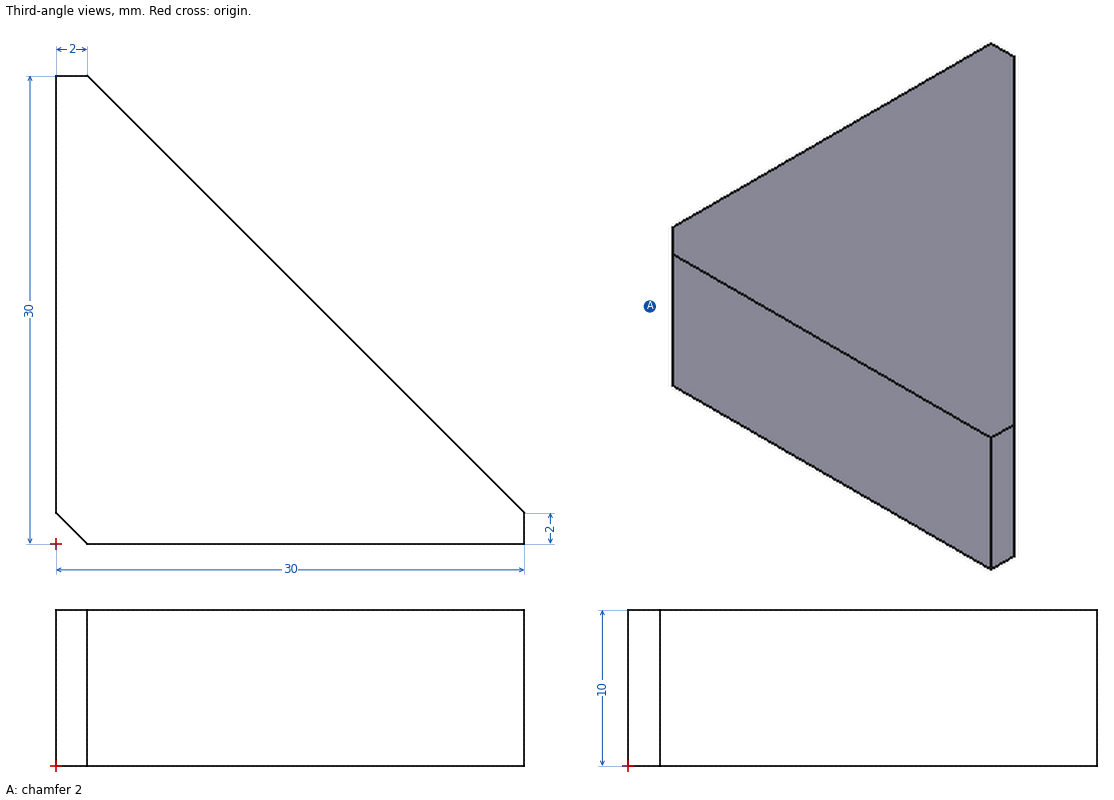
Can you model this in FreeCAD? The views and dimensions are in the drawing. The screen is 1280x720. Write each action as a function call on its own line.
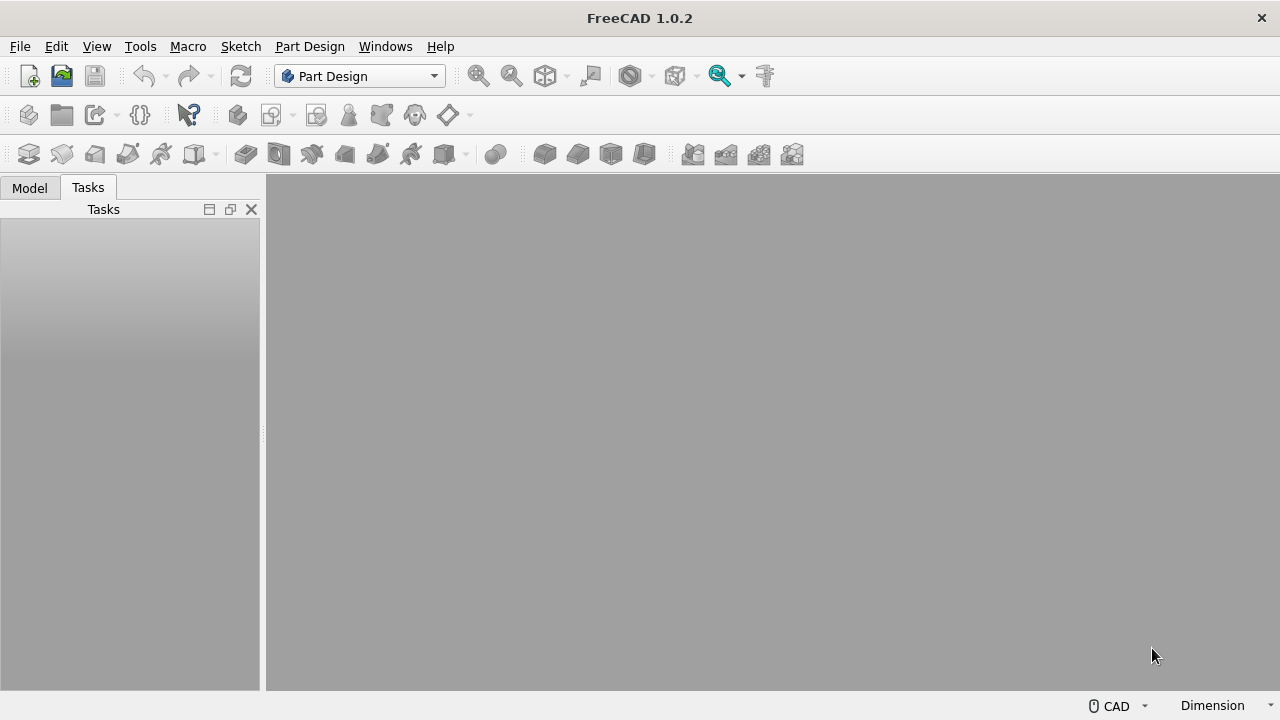
click(29, 76)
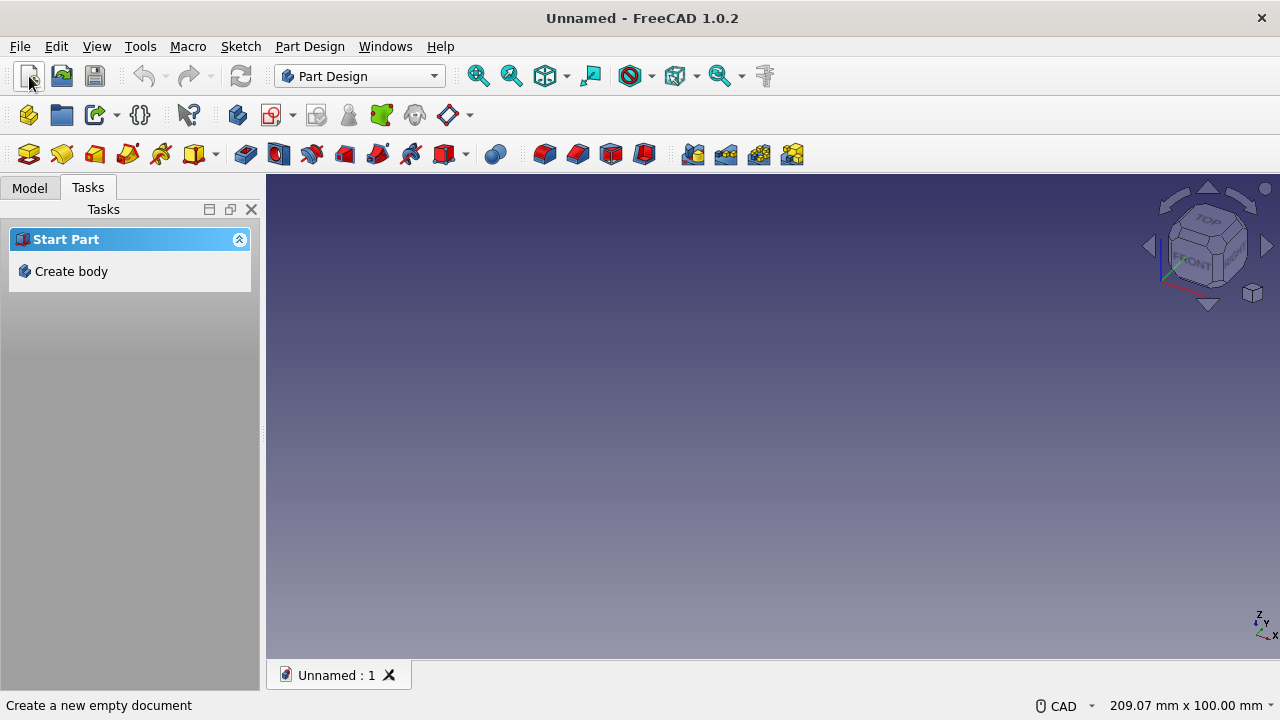
click(270, 116)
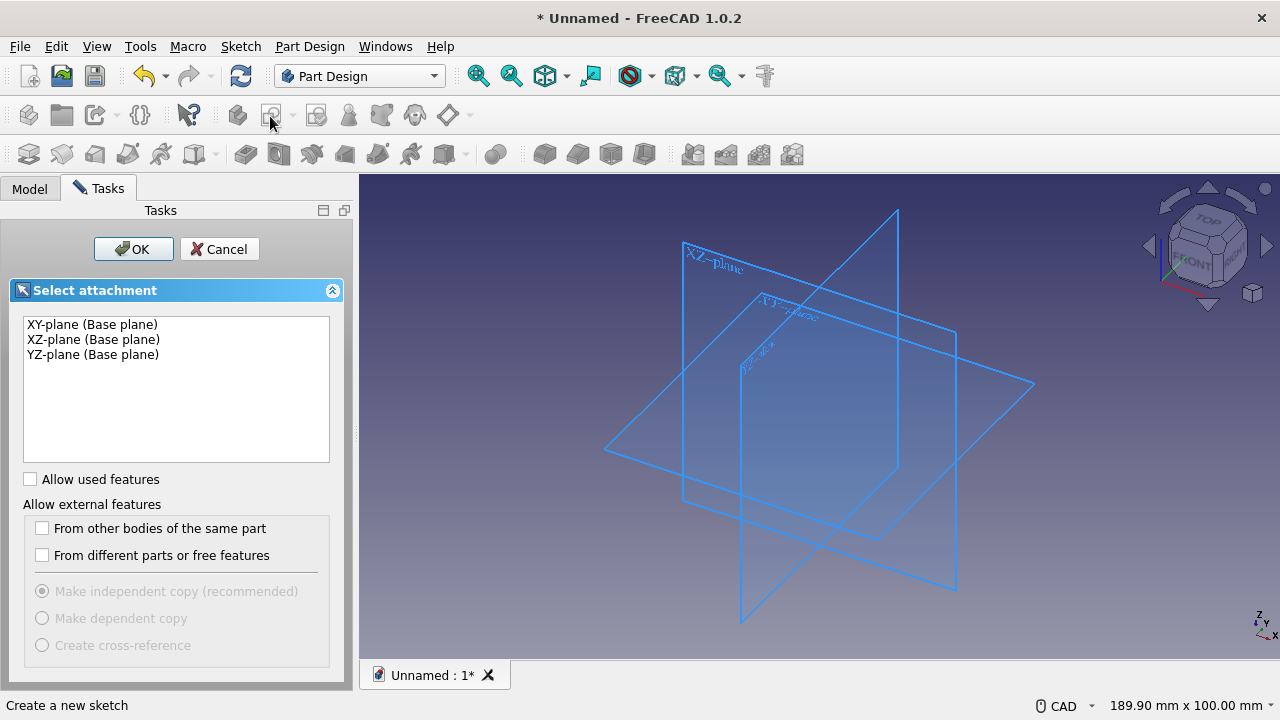
click(84, 324)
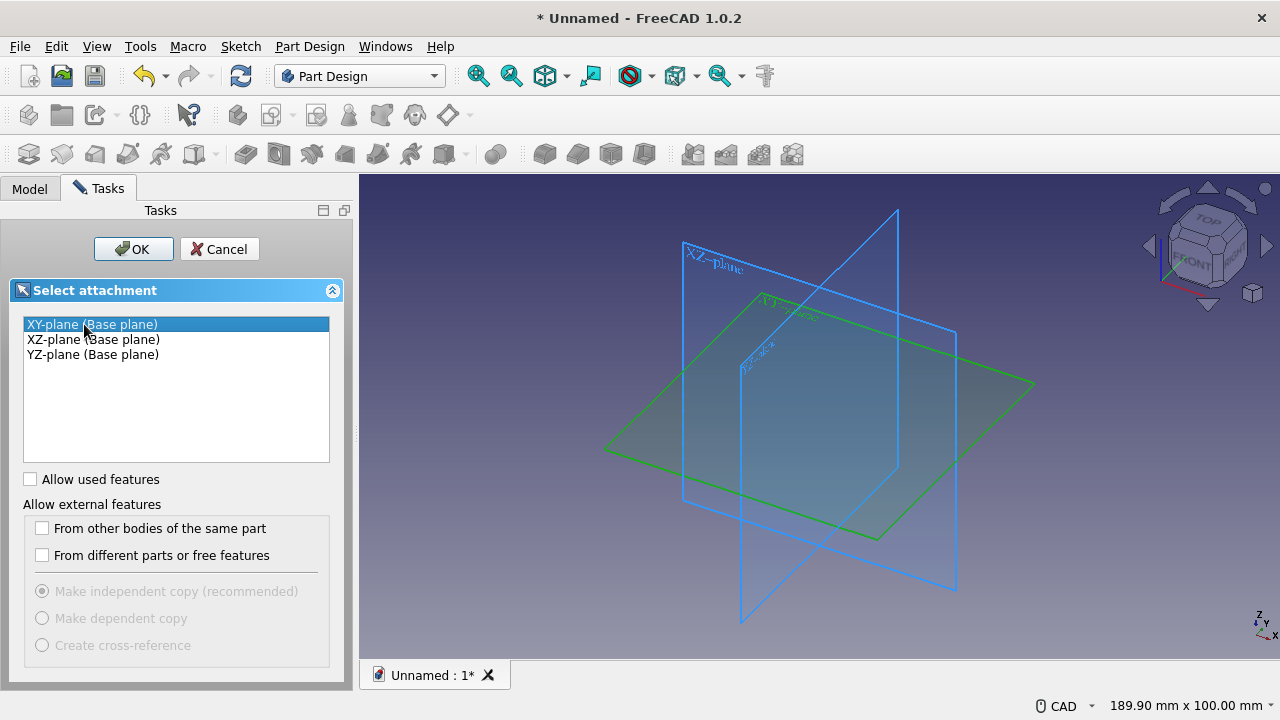
click(134, 249)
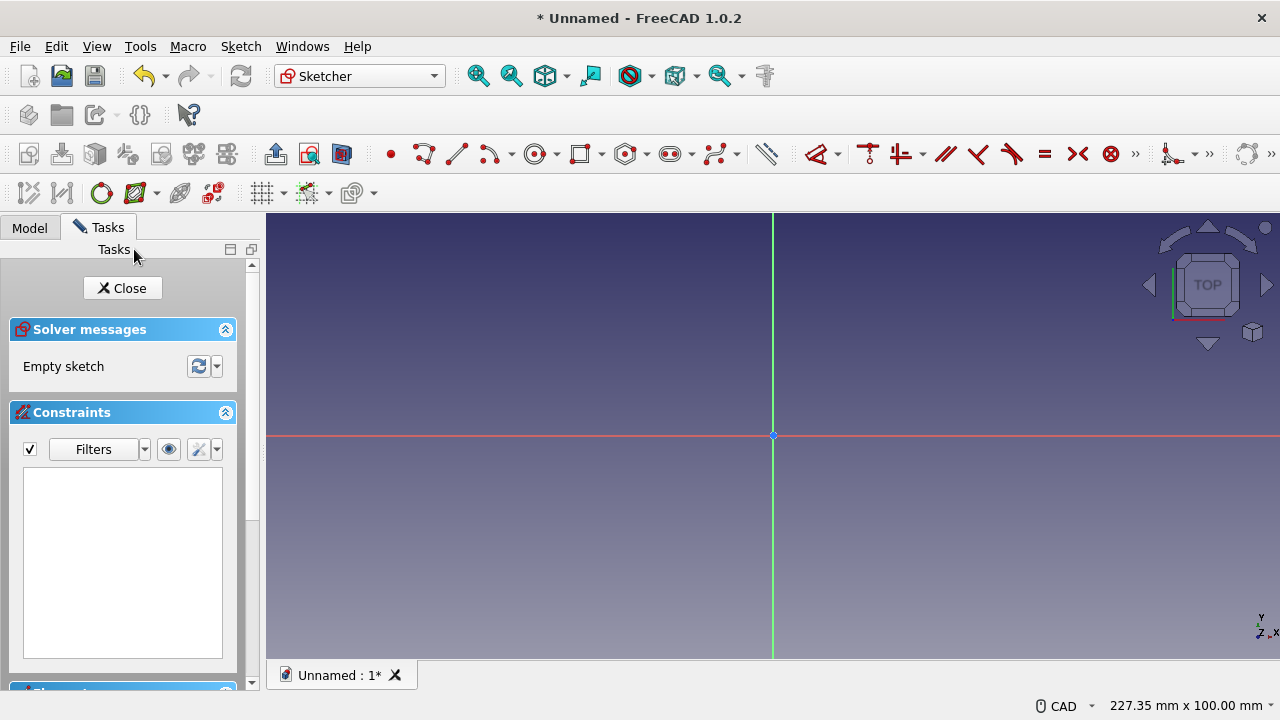
scroll(950, 315, up, 4)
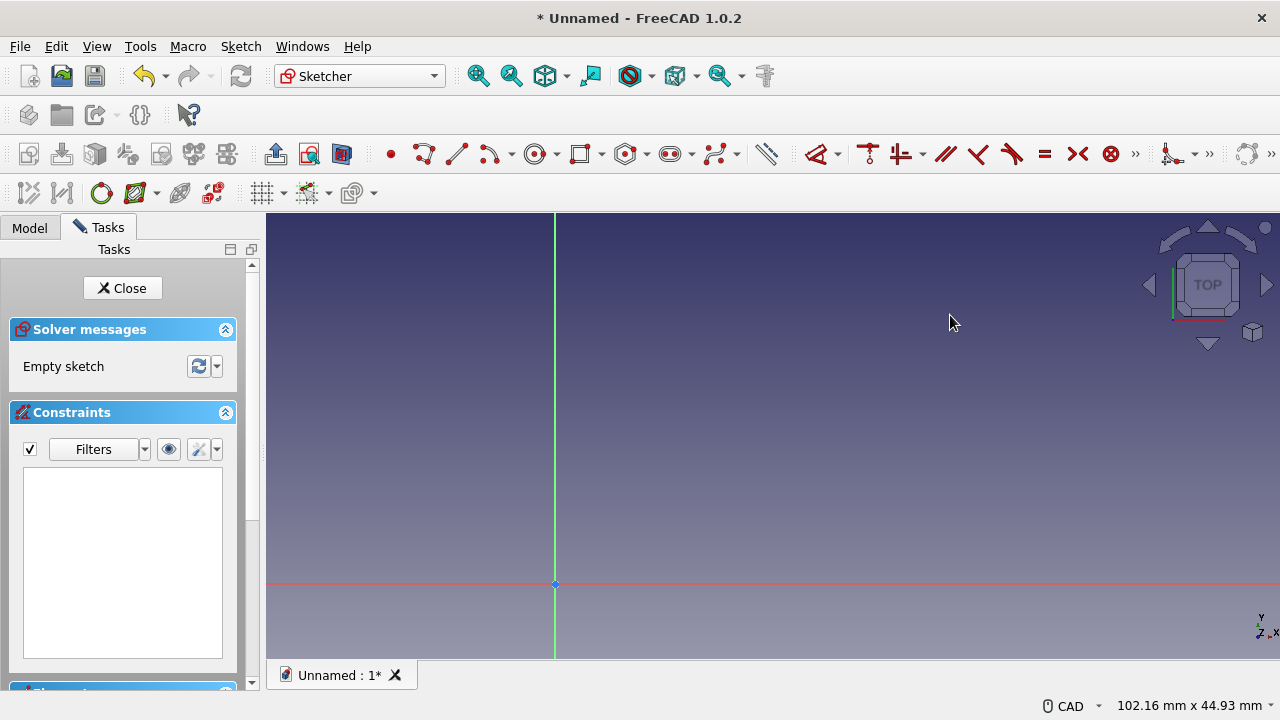
click(424, 154)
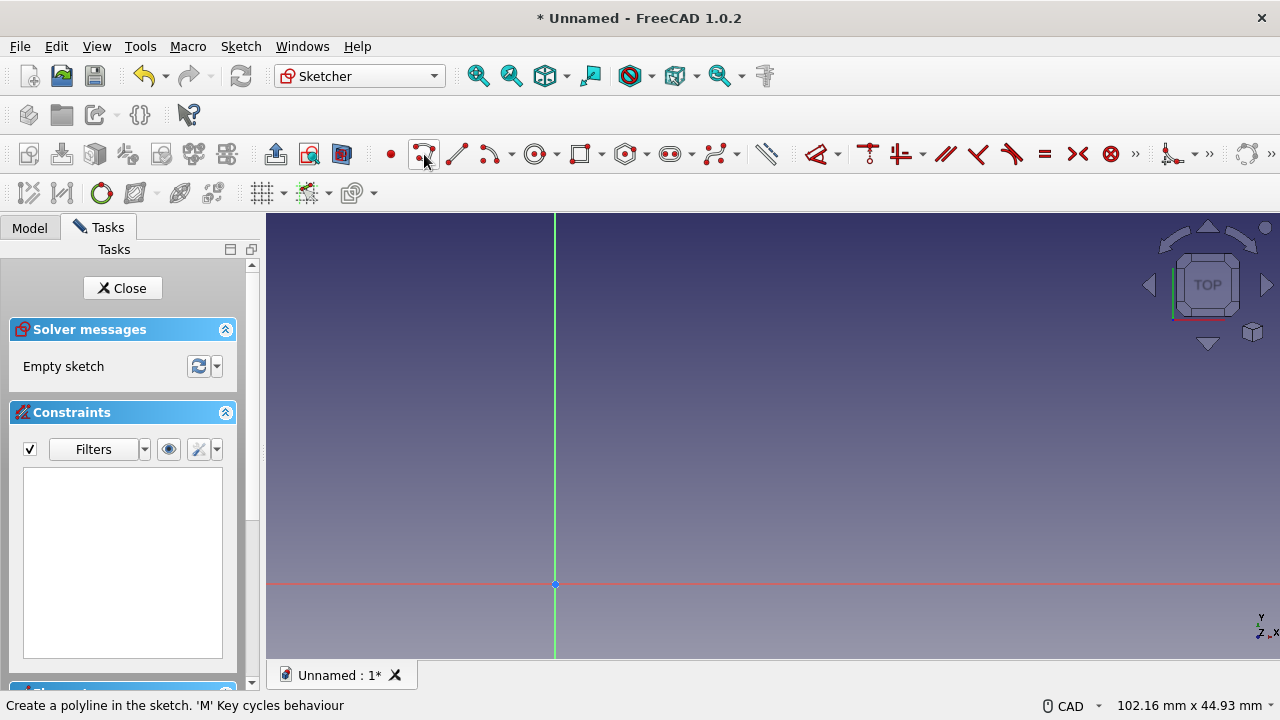
click(555, 584)
click(853, 575)
click(853, 564)
click(575, 286)
click(564, 286)
click(555, 584)
key(Escape)
key(Escape)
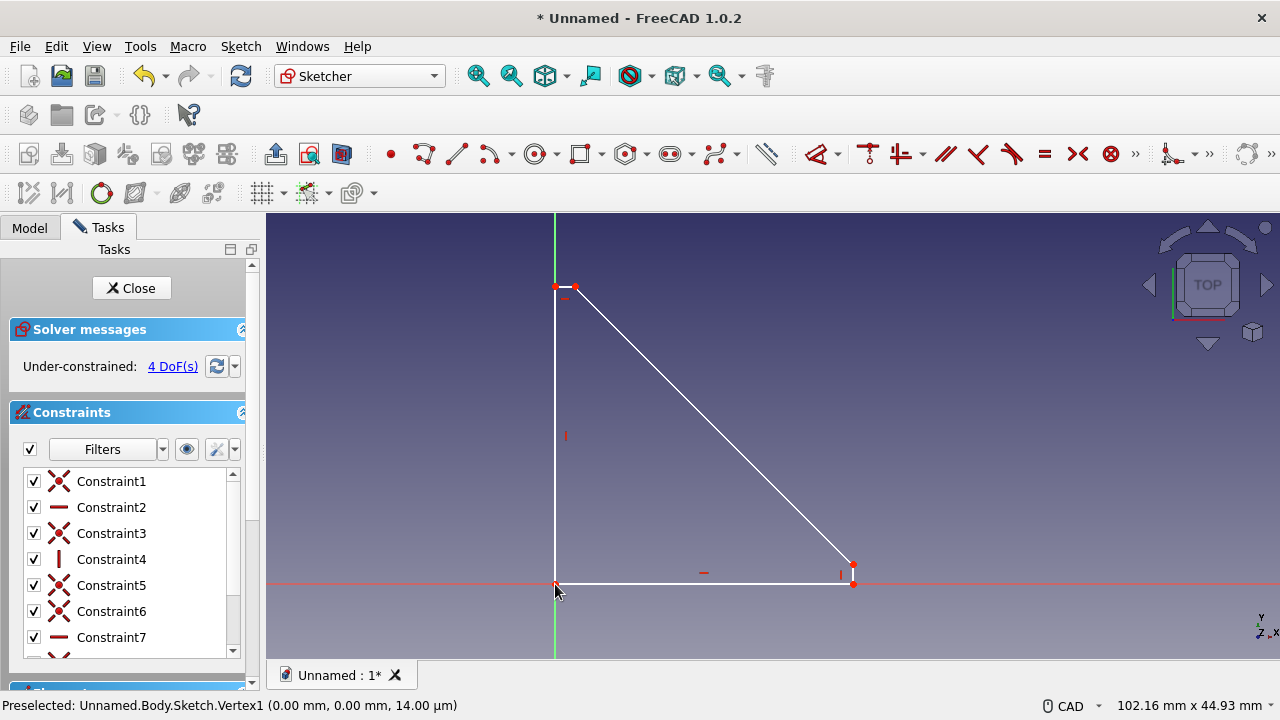
click(816, 154)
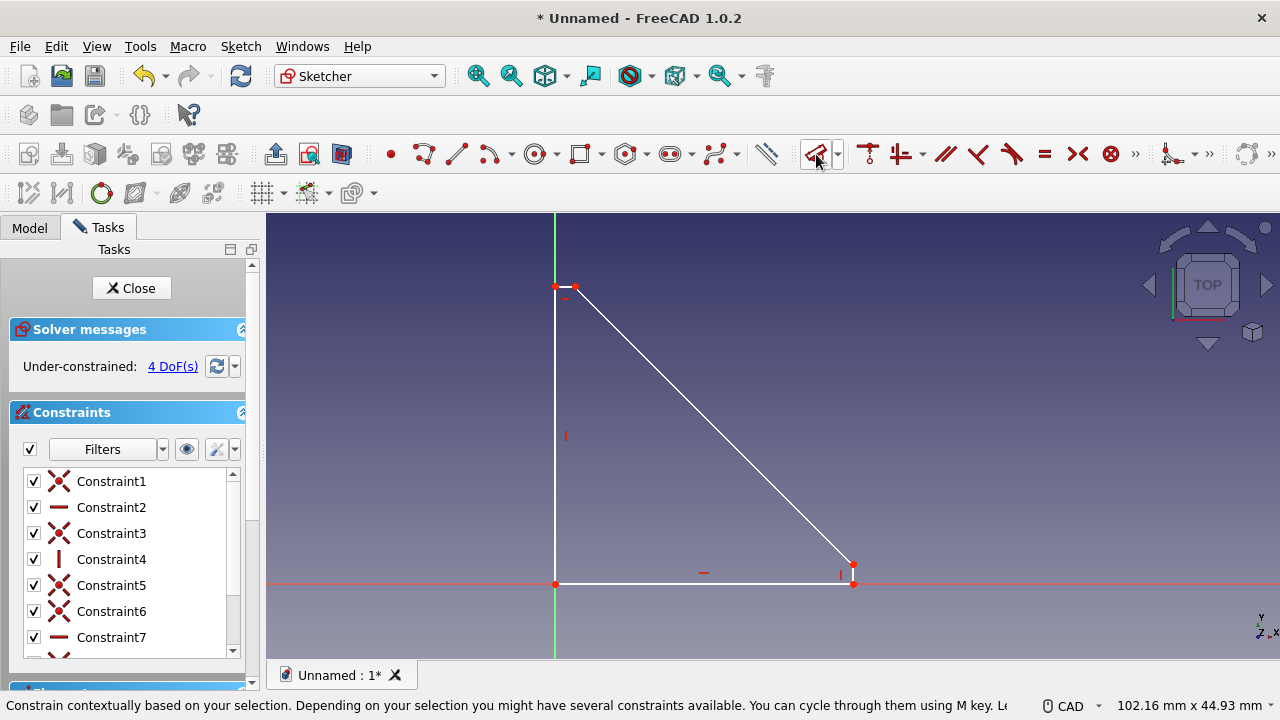
scroll(853, 575, up, 4)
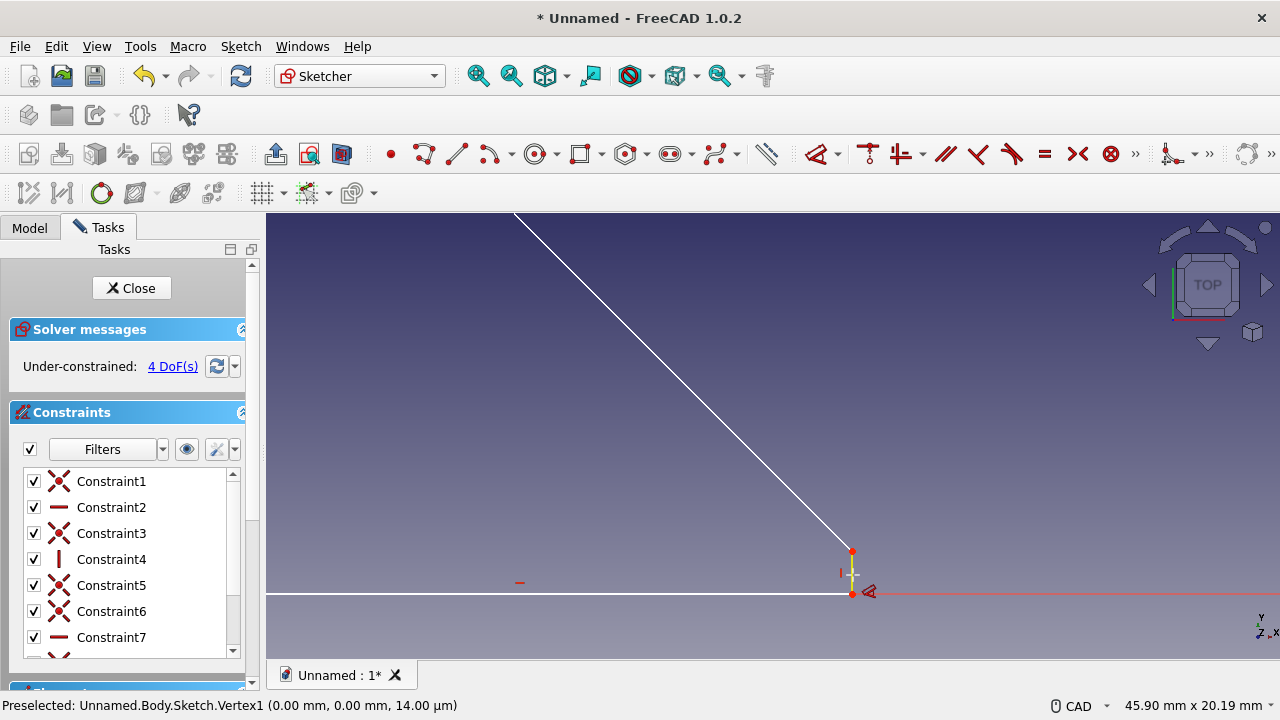
click(852, 573)
click(886, 573)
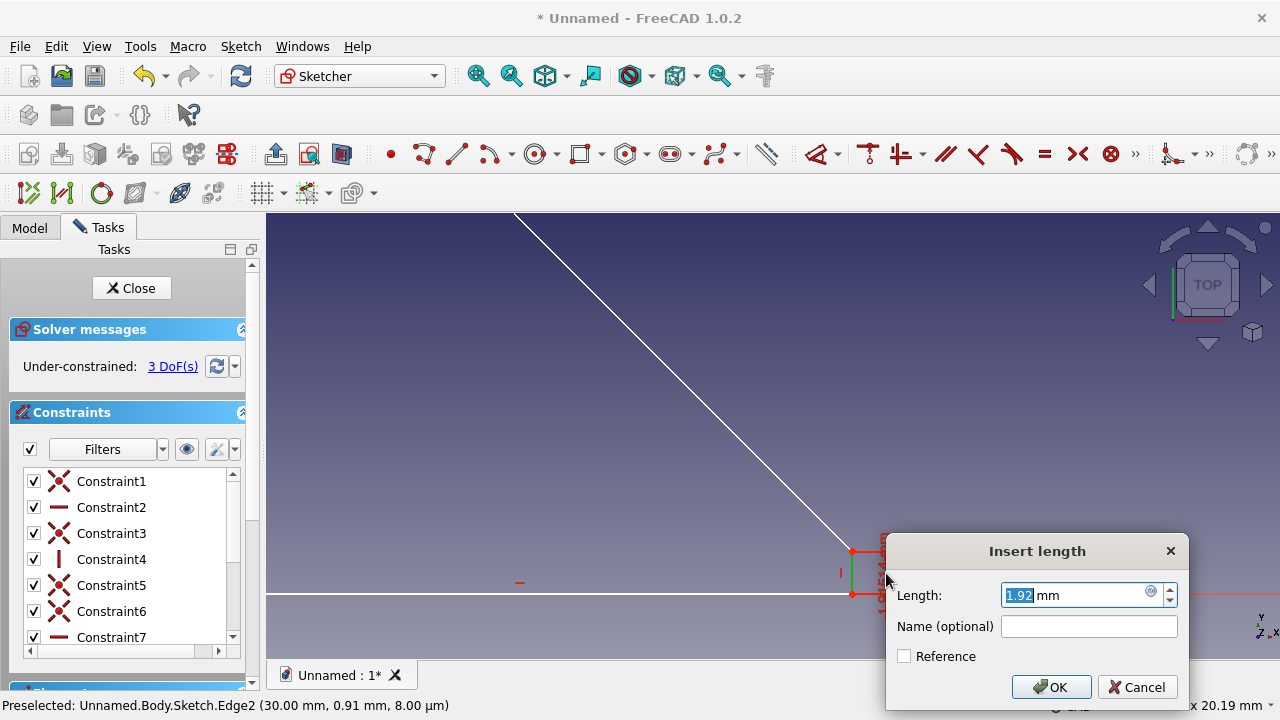
text(2)
key(Return)